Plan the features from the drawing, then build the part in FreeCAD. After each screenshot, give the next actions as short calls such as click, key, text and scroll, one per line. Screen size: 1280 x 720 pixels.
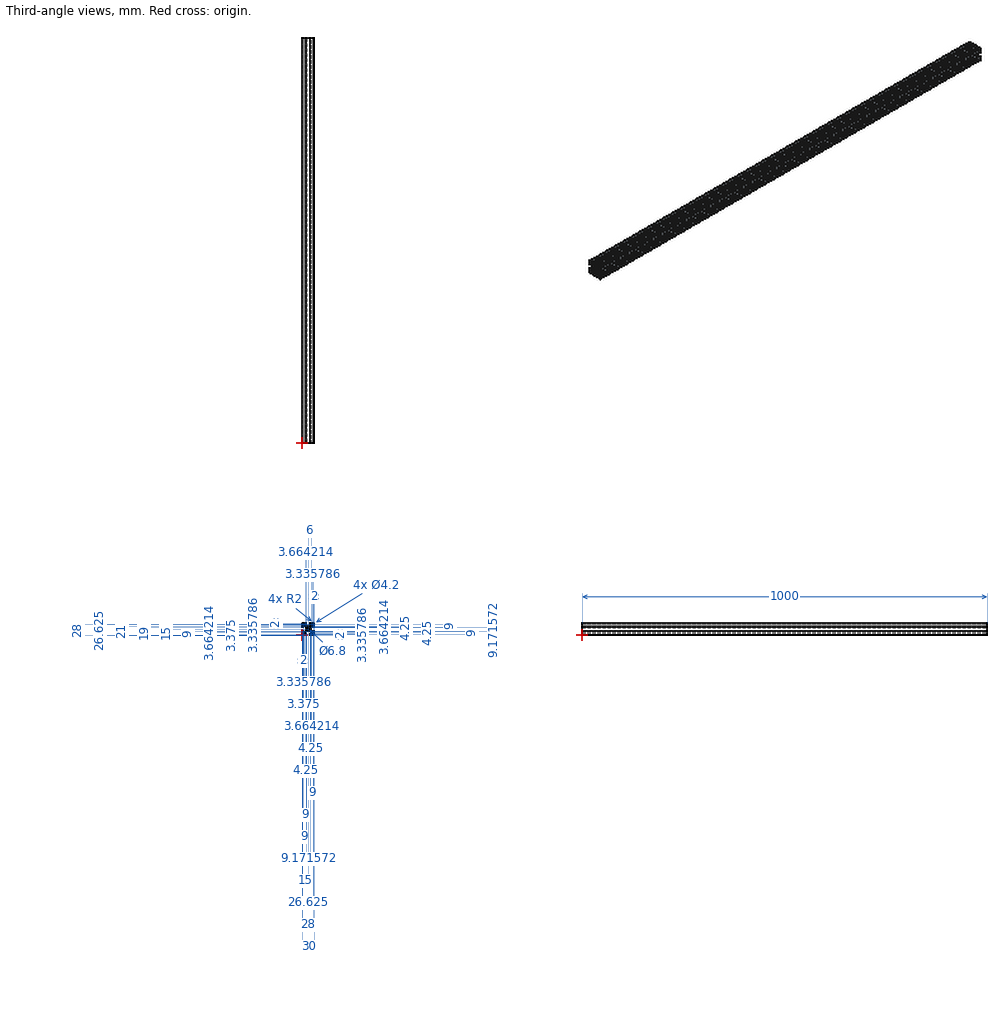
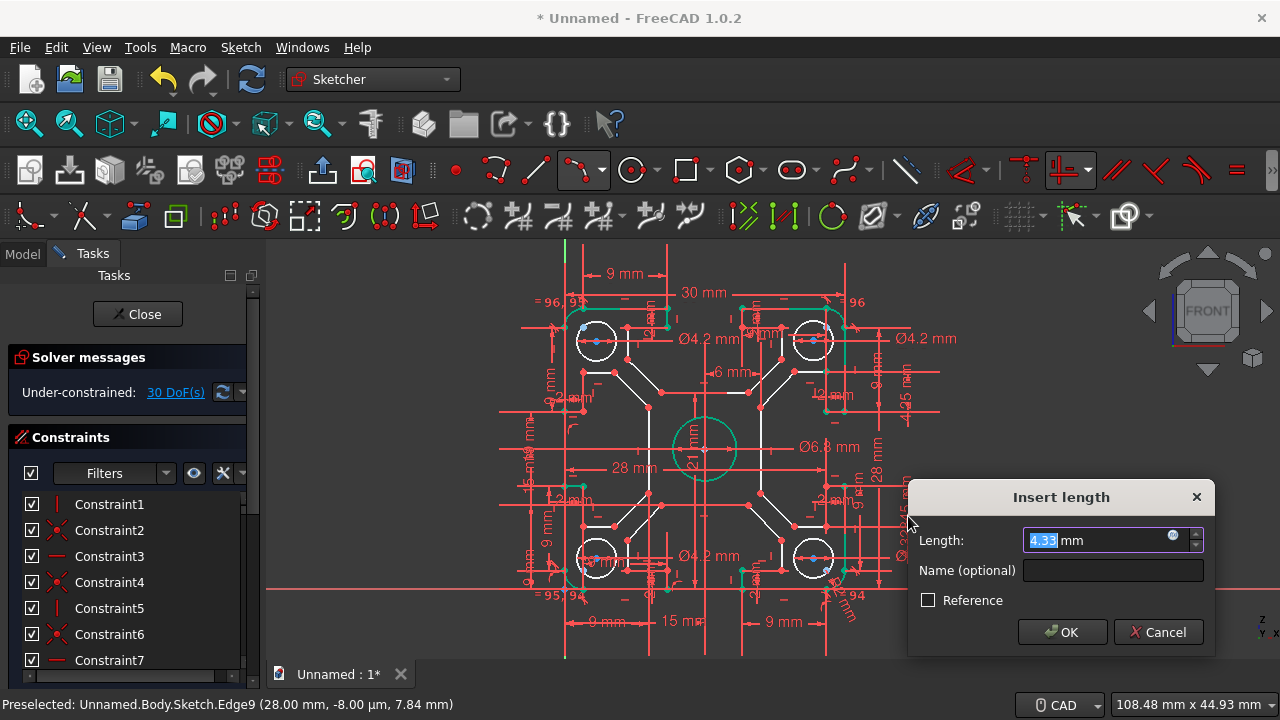
text(4.25)
key(Return)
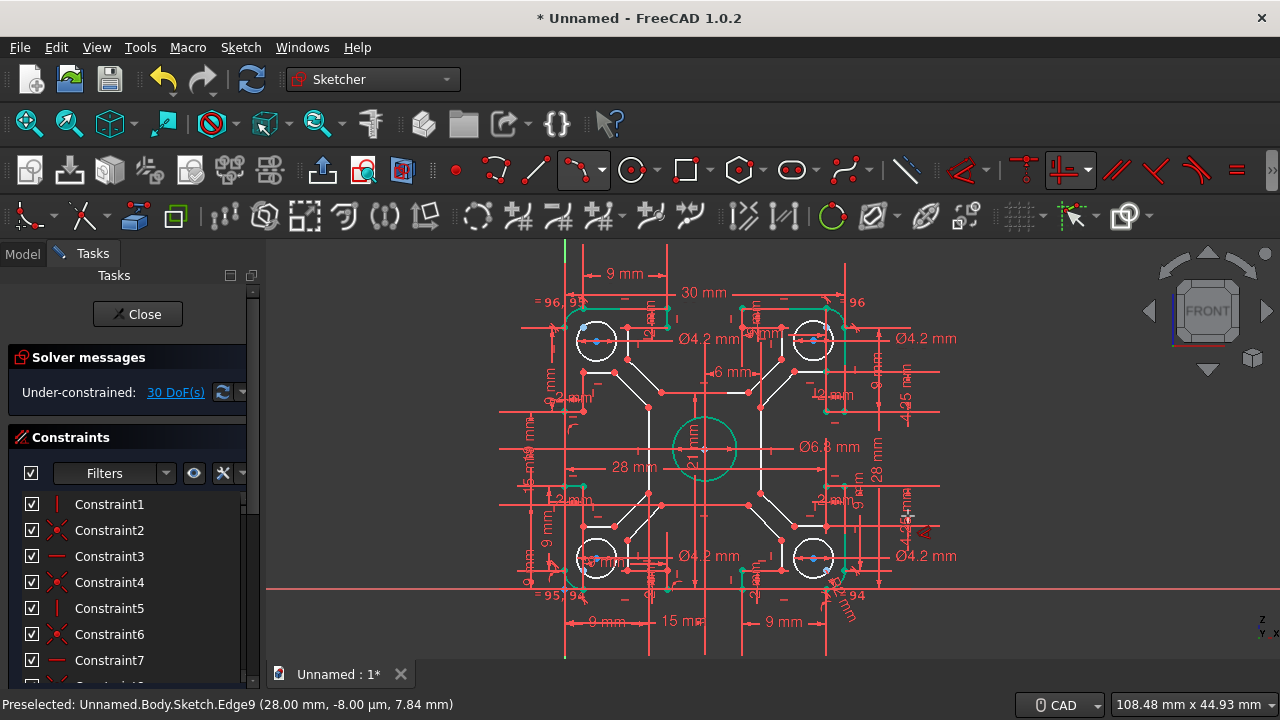
click(754, 571)
click(753, 537)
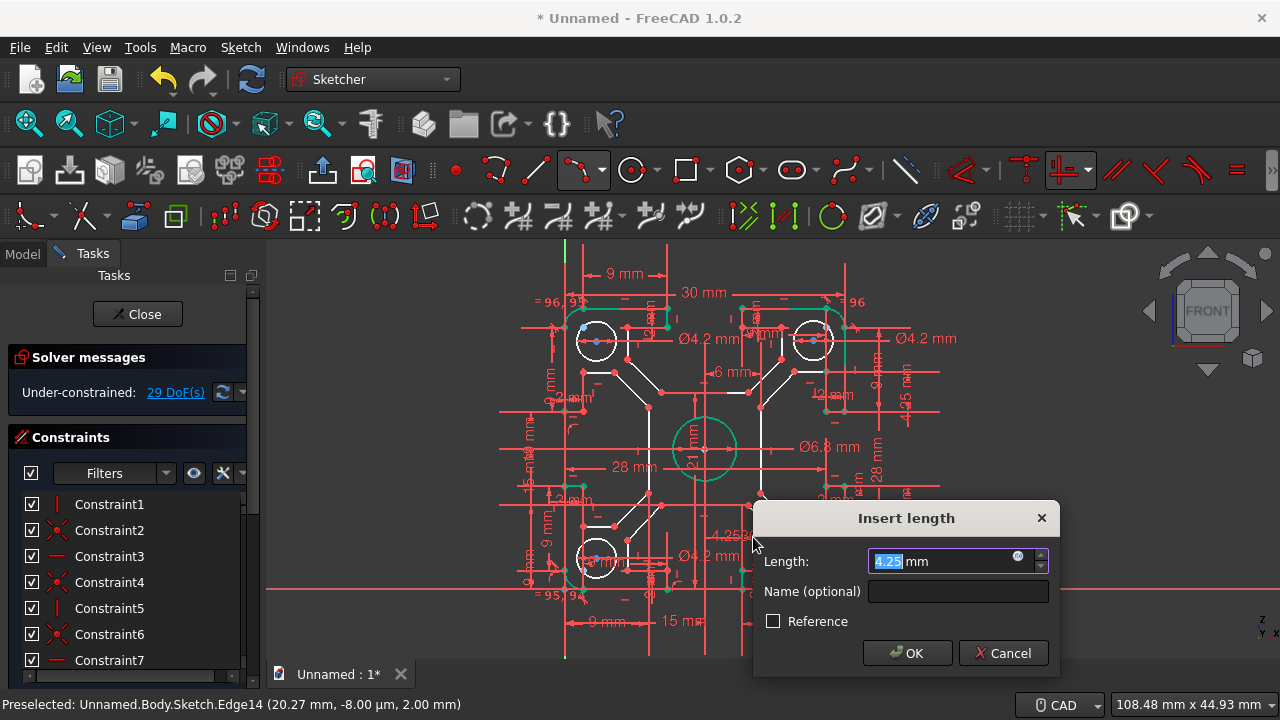
text(4.25)
key(Return)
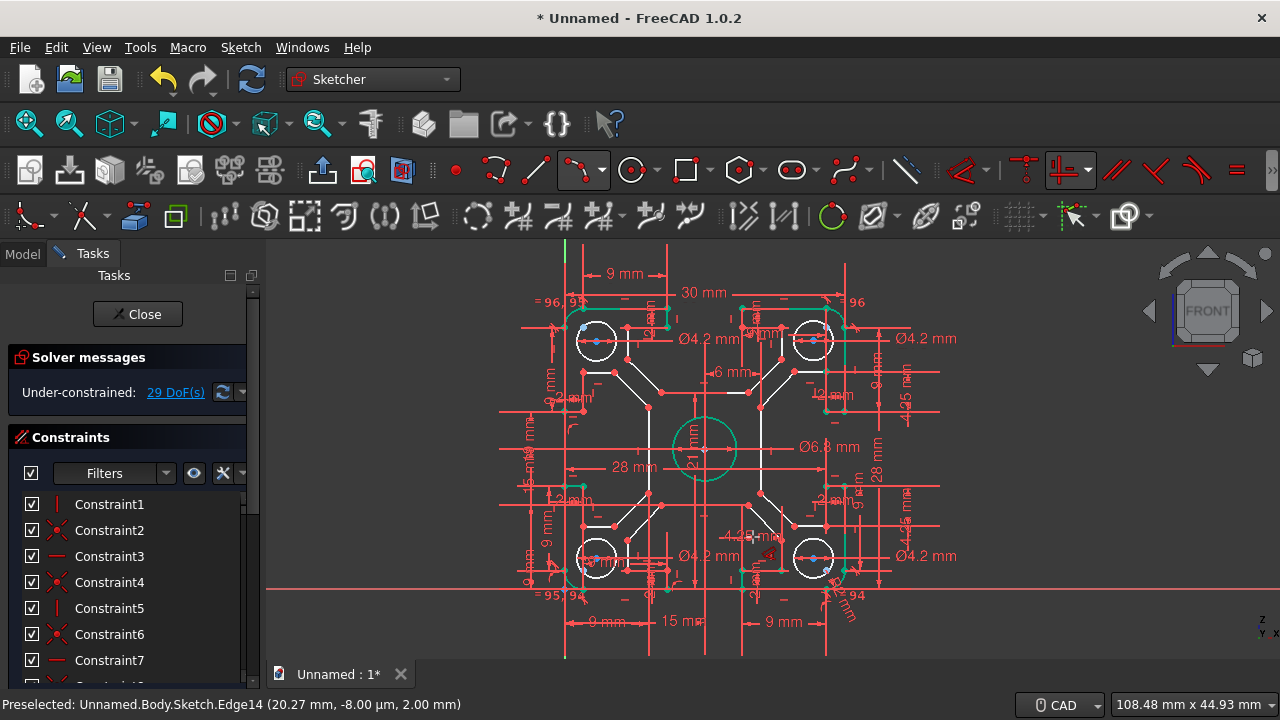
click(640, 571)
click(657, 537)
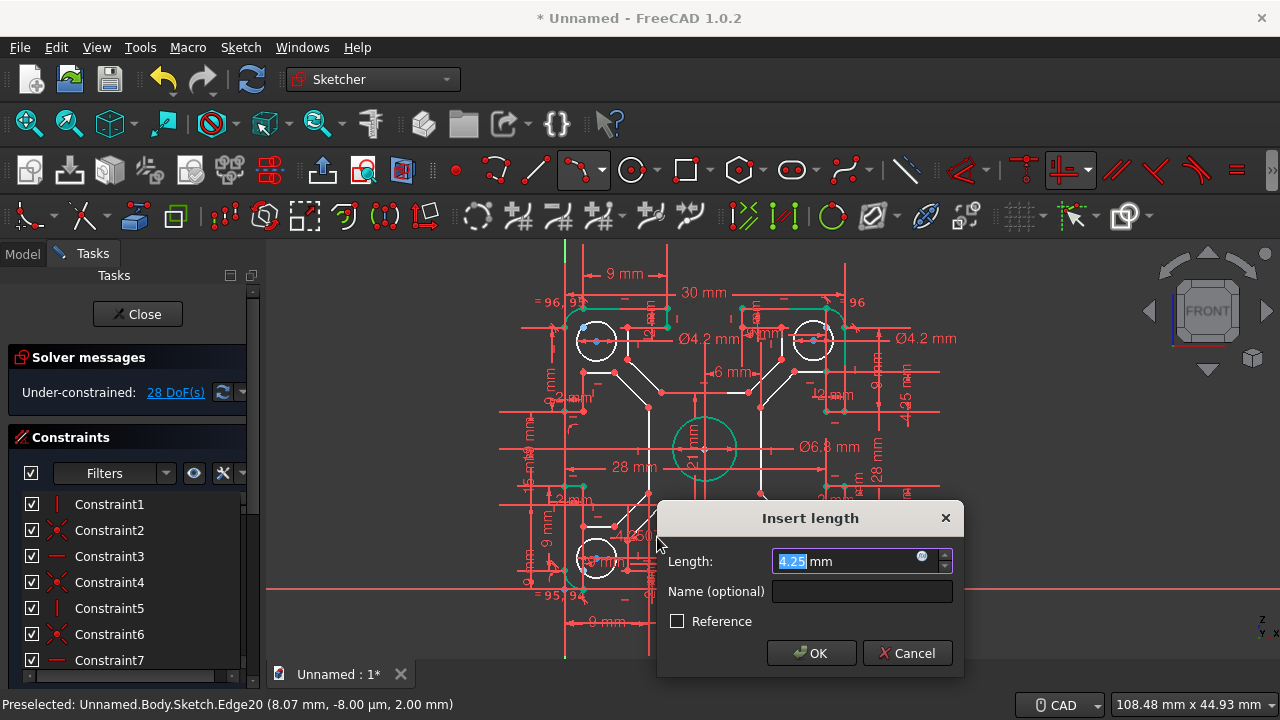
text(4.25)
key(Return)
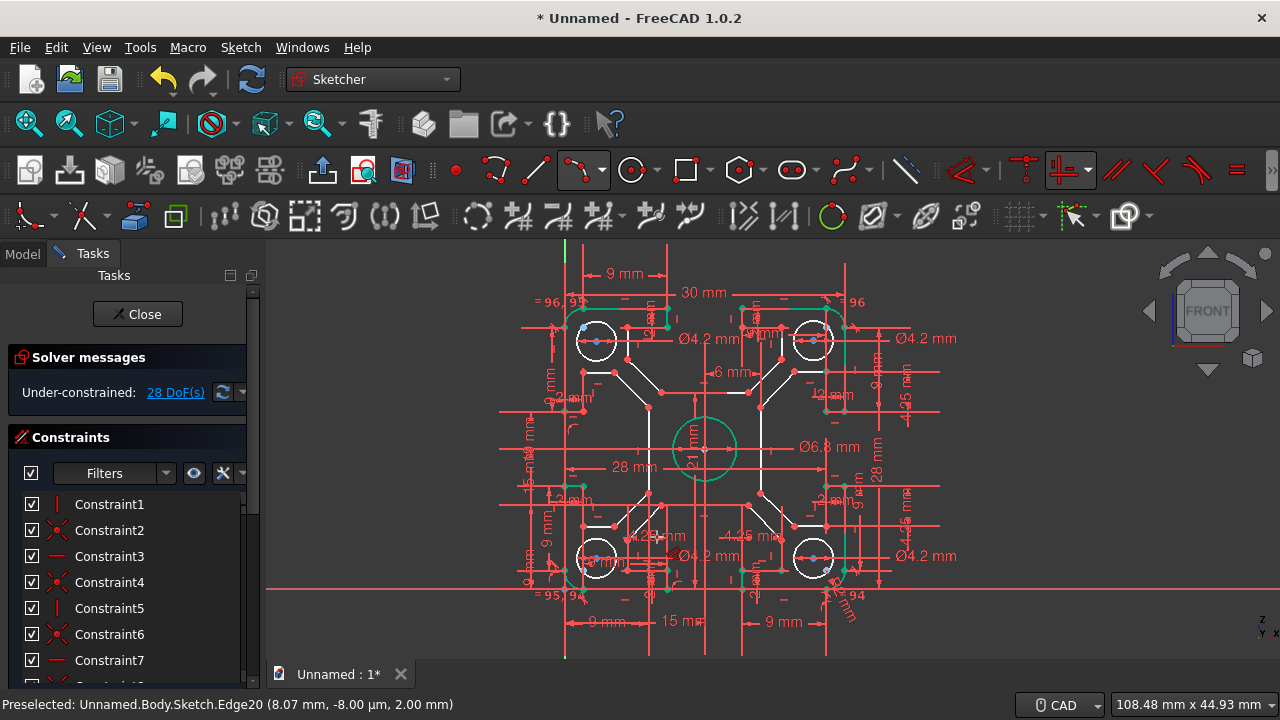
click(583, 499)
click(501, 507)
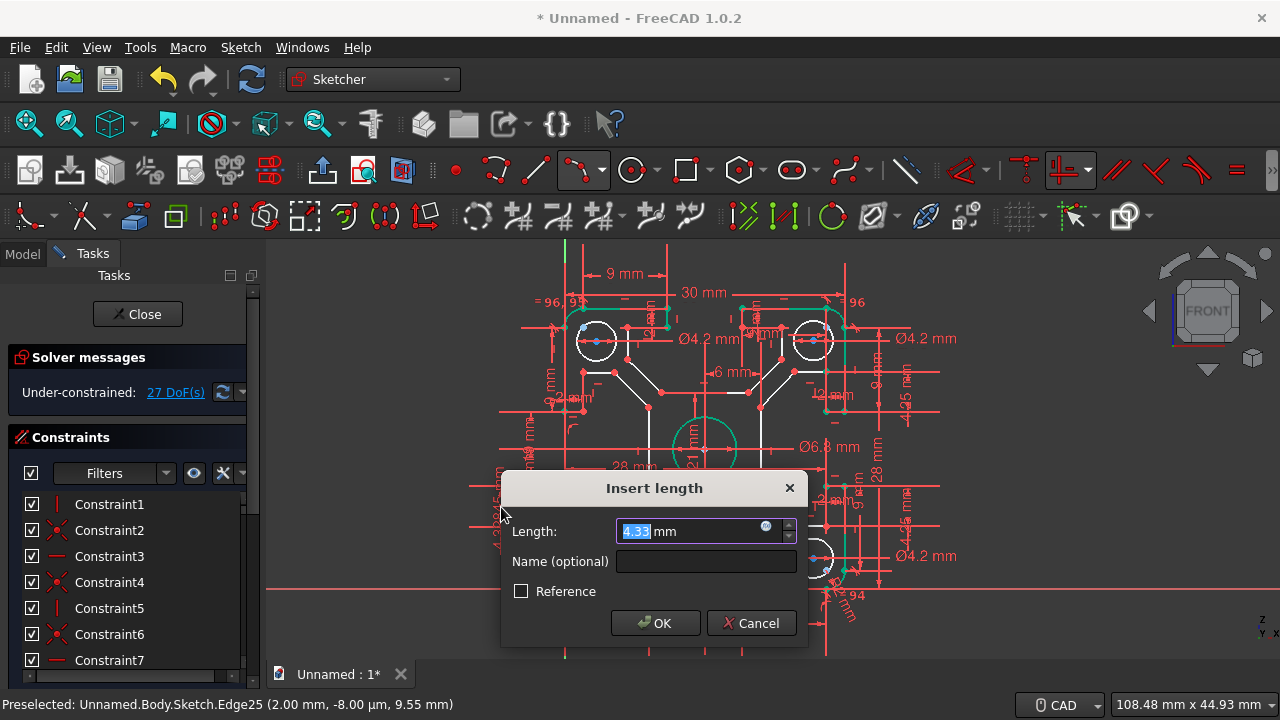
text(4.25)
key(Return)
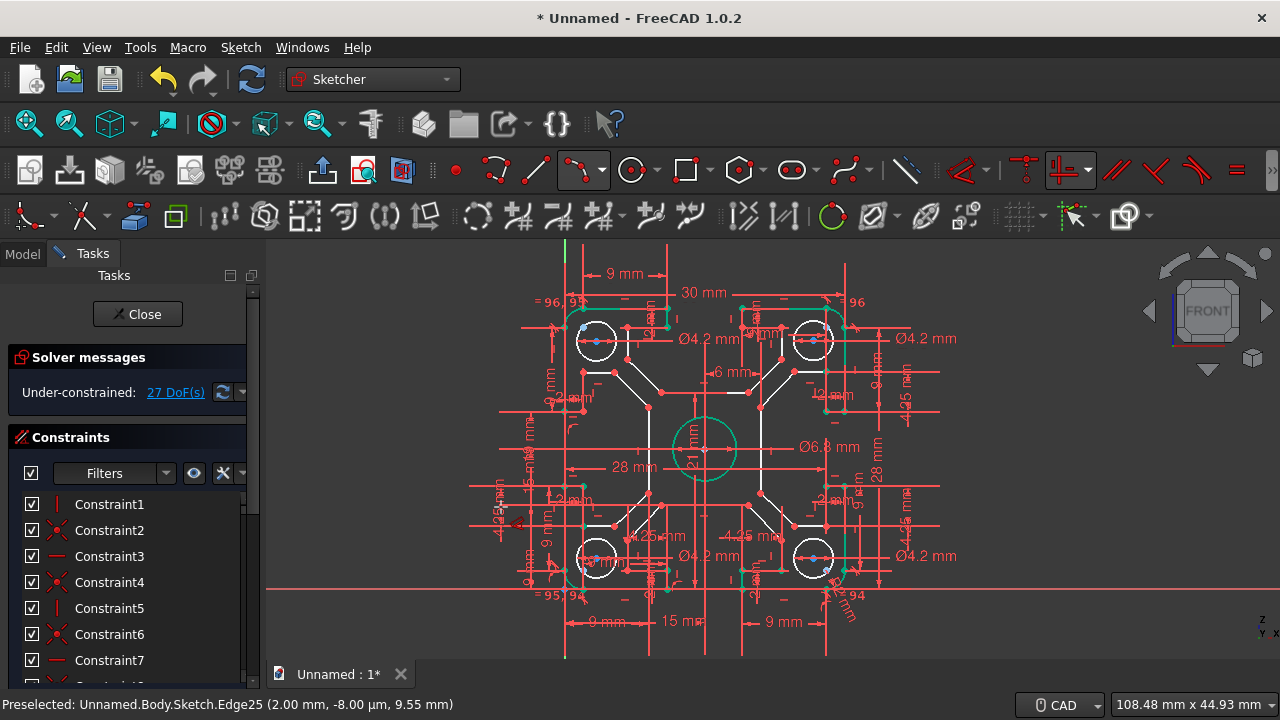
click(583, 384)
click(501, 406)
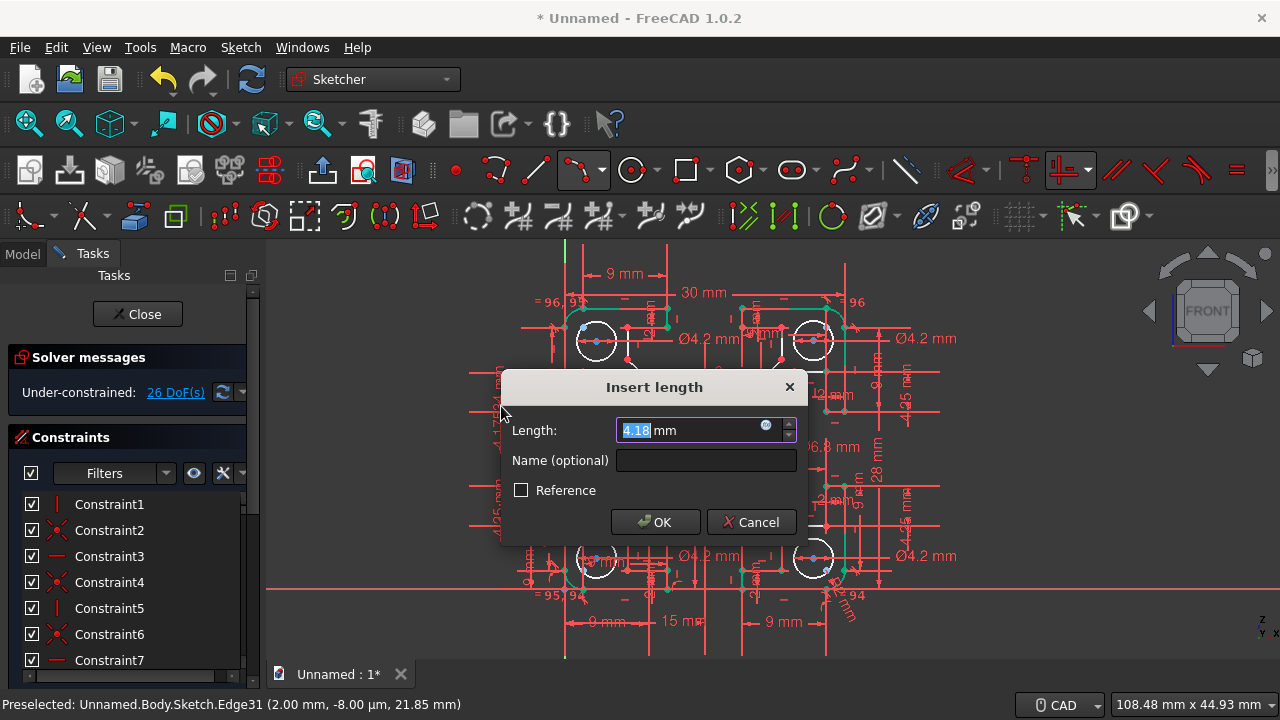
text(4.25)
key(Return)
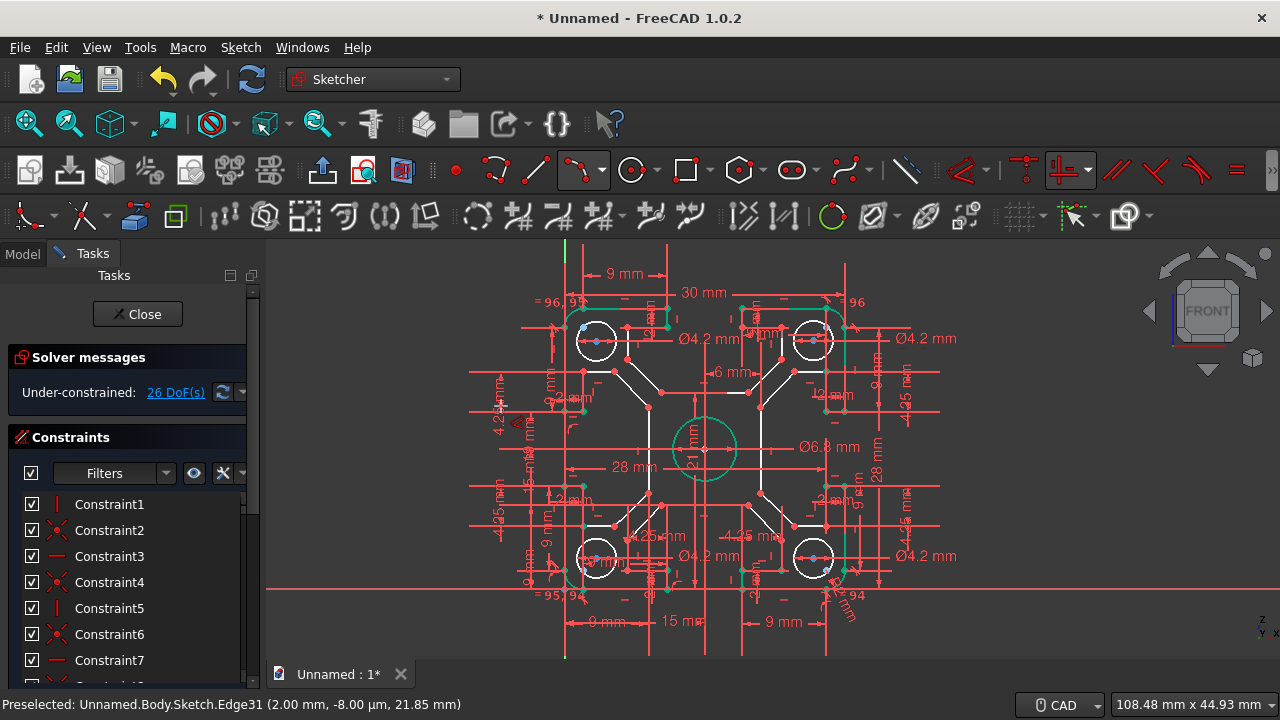
click(655, 328)
click(657, 362)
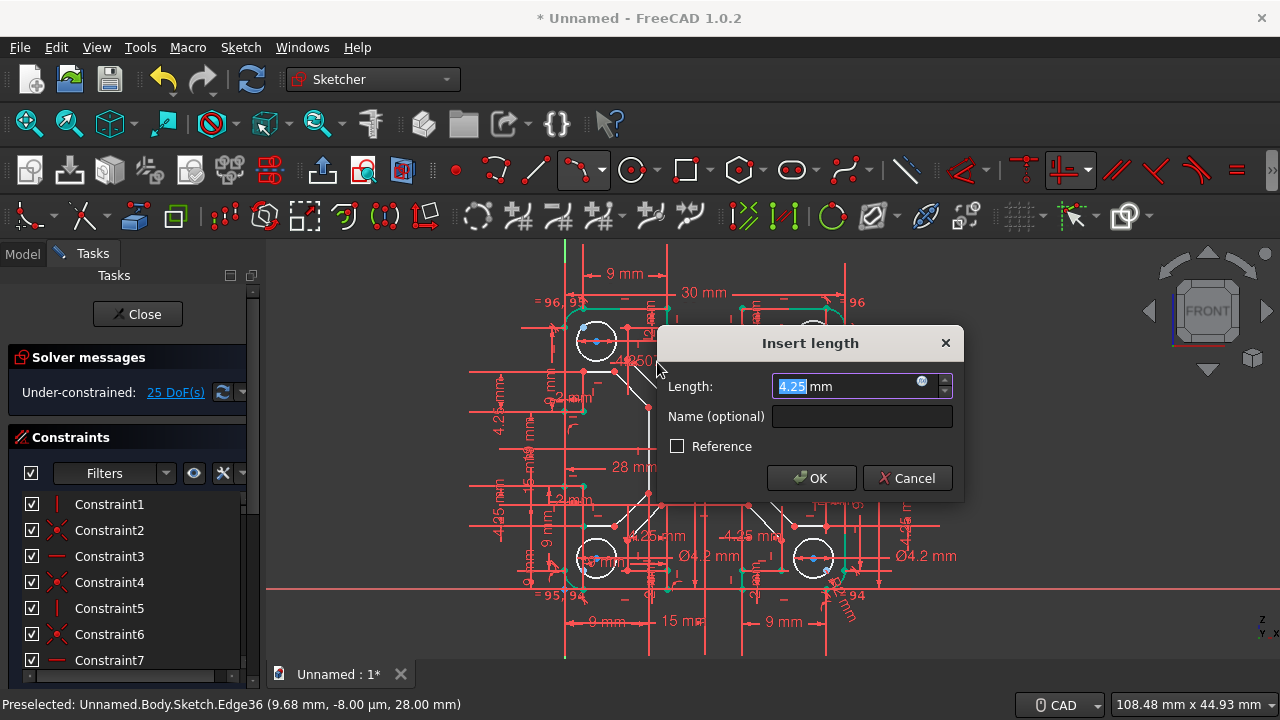
text(4.25)
key(Return)